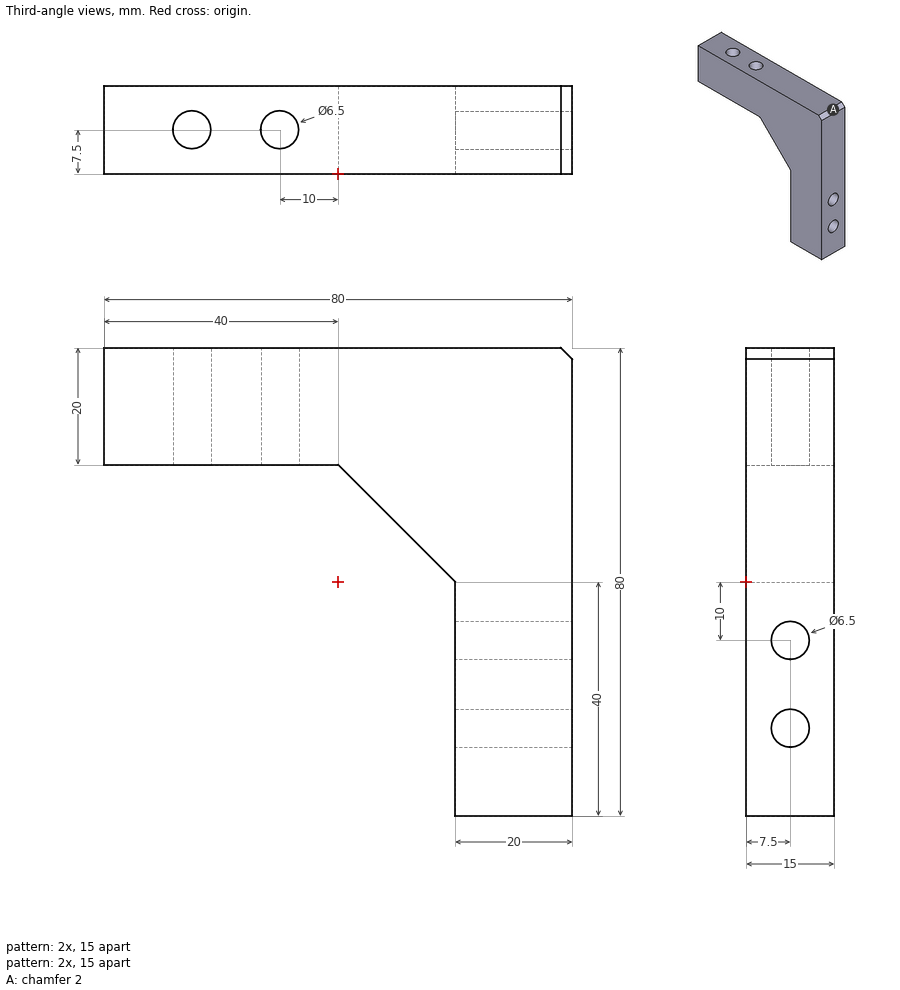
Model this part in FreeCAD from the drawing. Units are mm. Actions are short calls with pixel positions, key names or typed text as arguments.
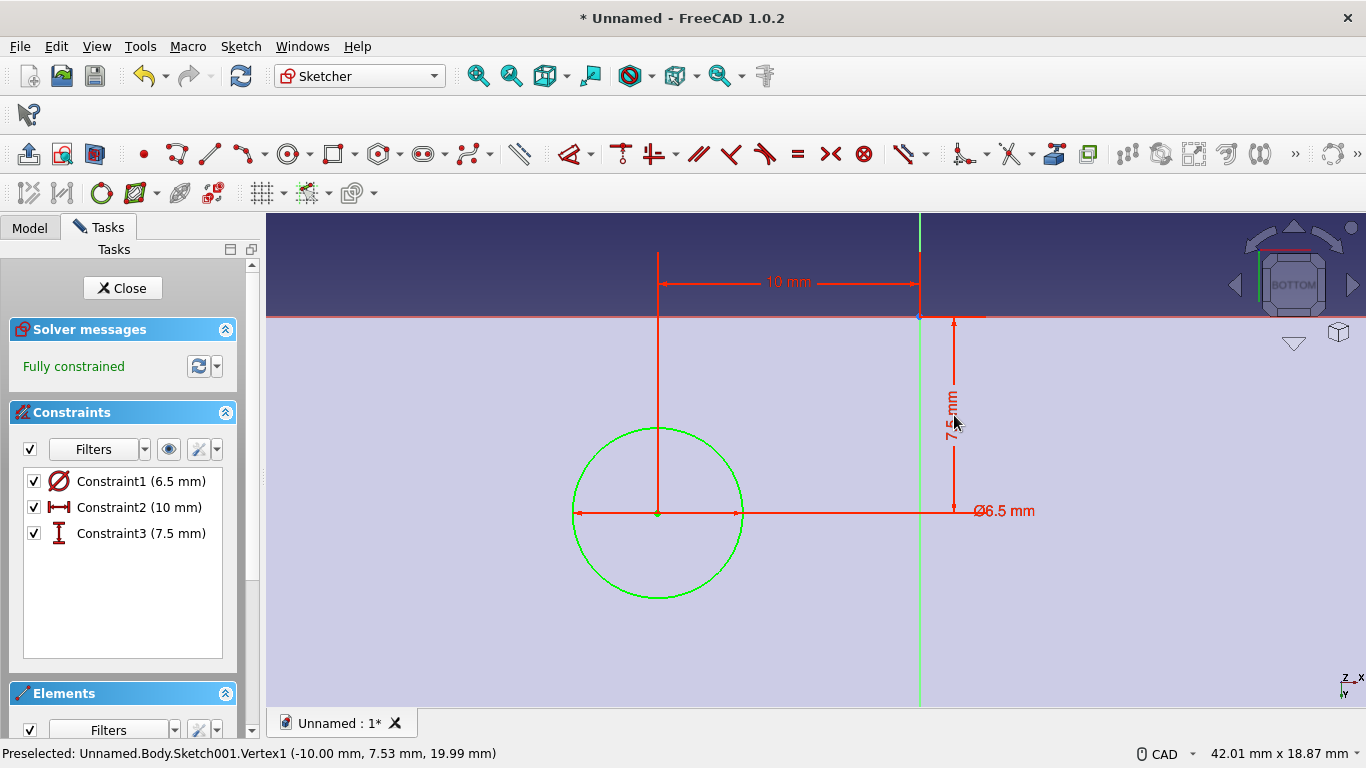
click(123, 288)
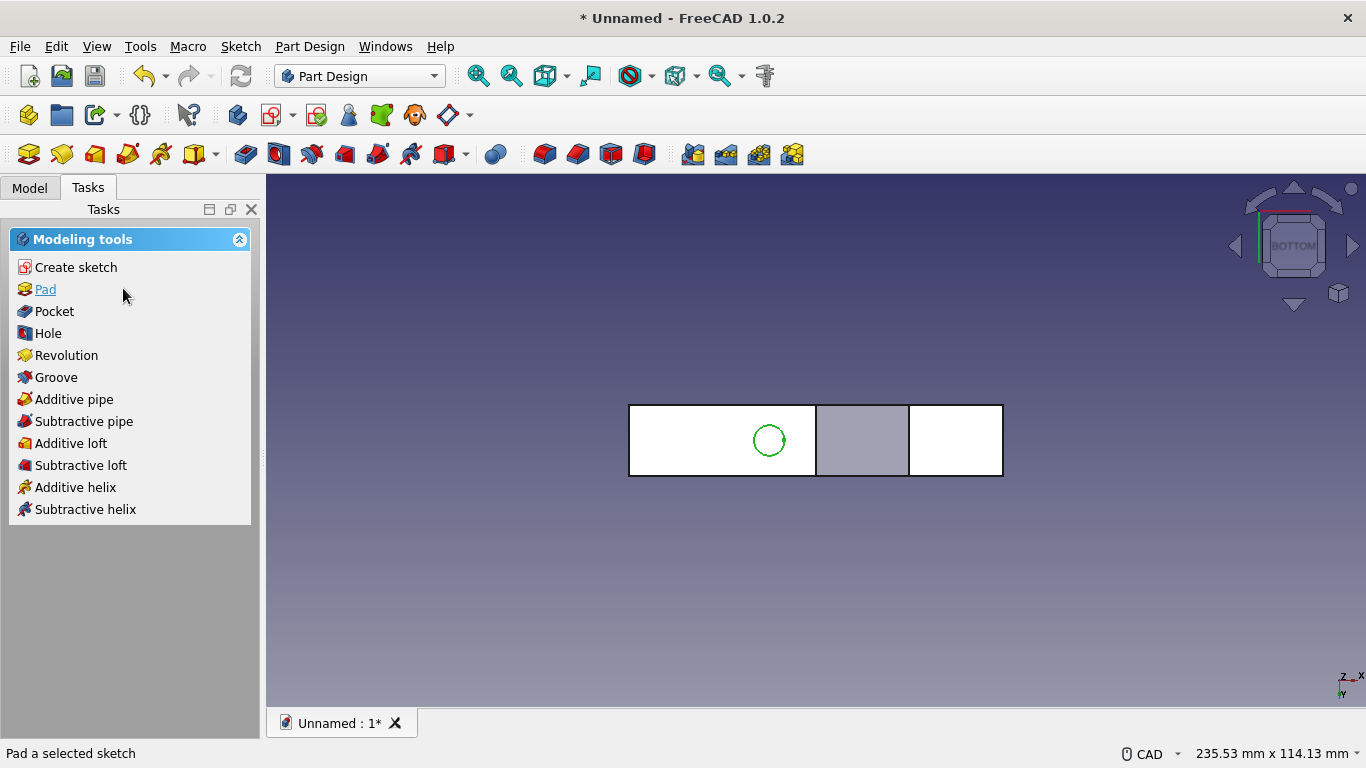
click(246, 154)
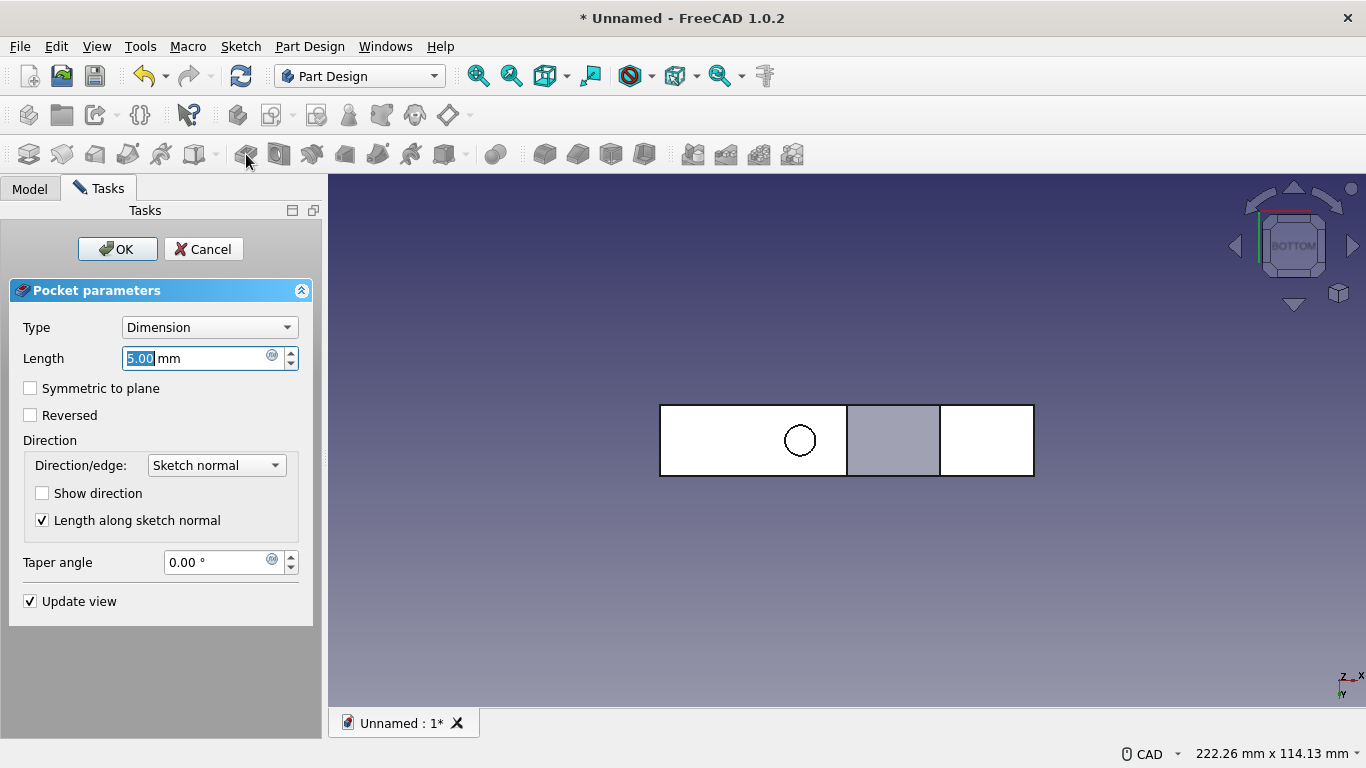
click(210, 328)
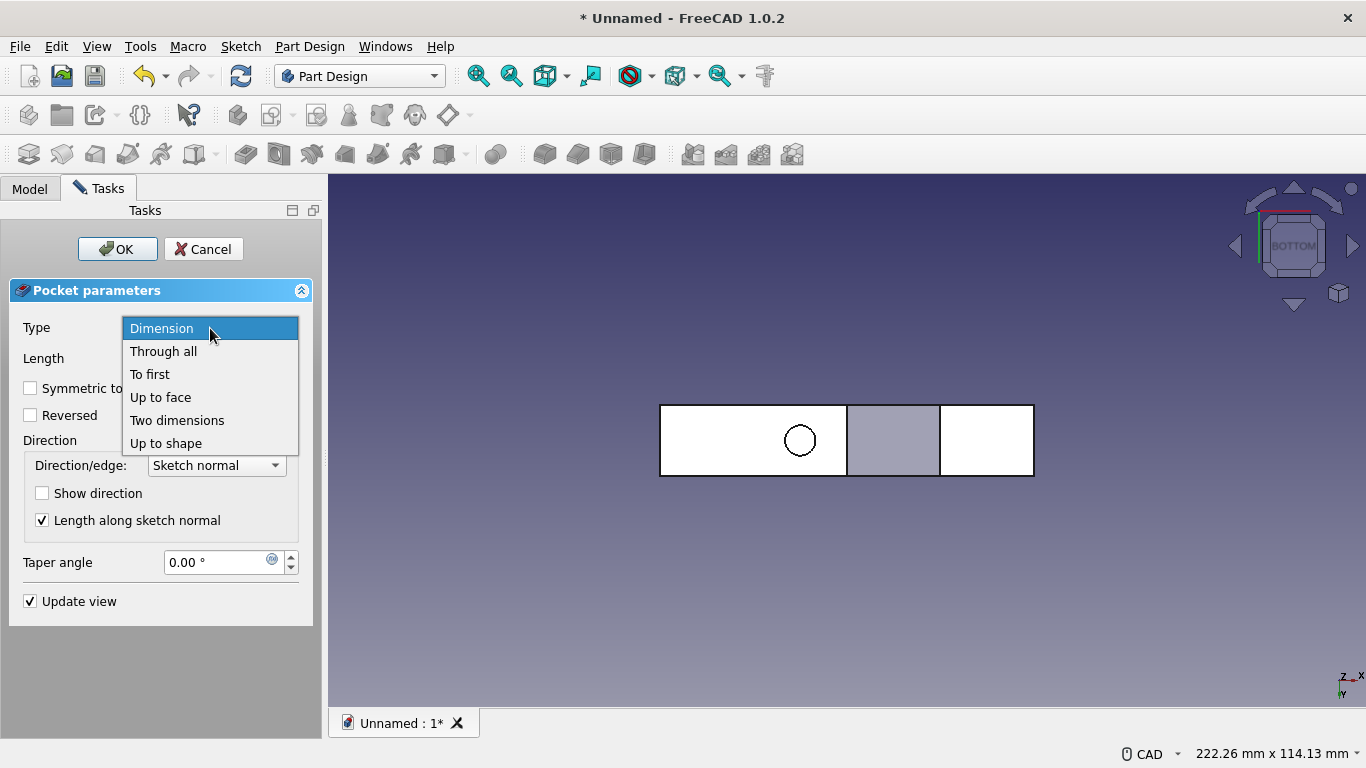
click(208, 352)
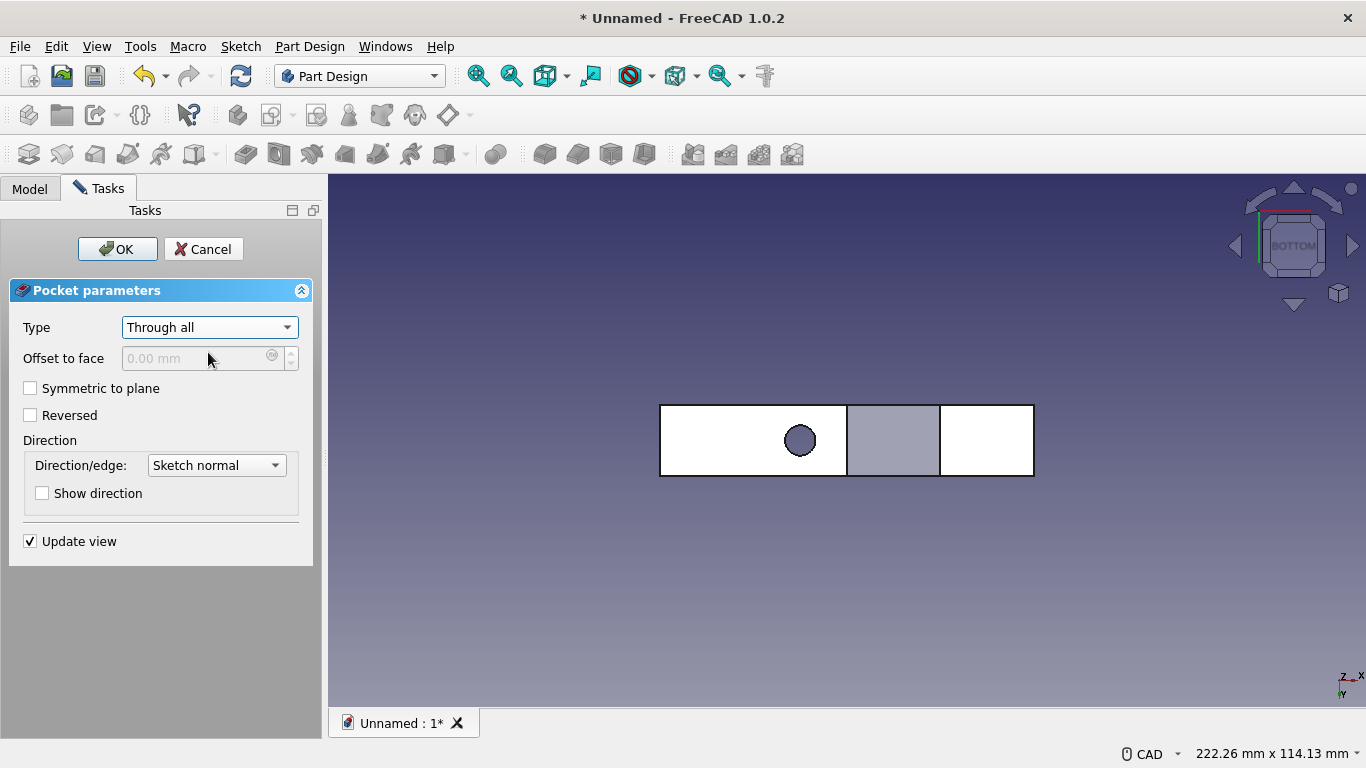
click(118, 249)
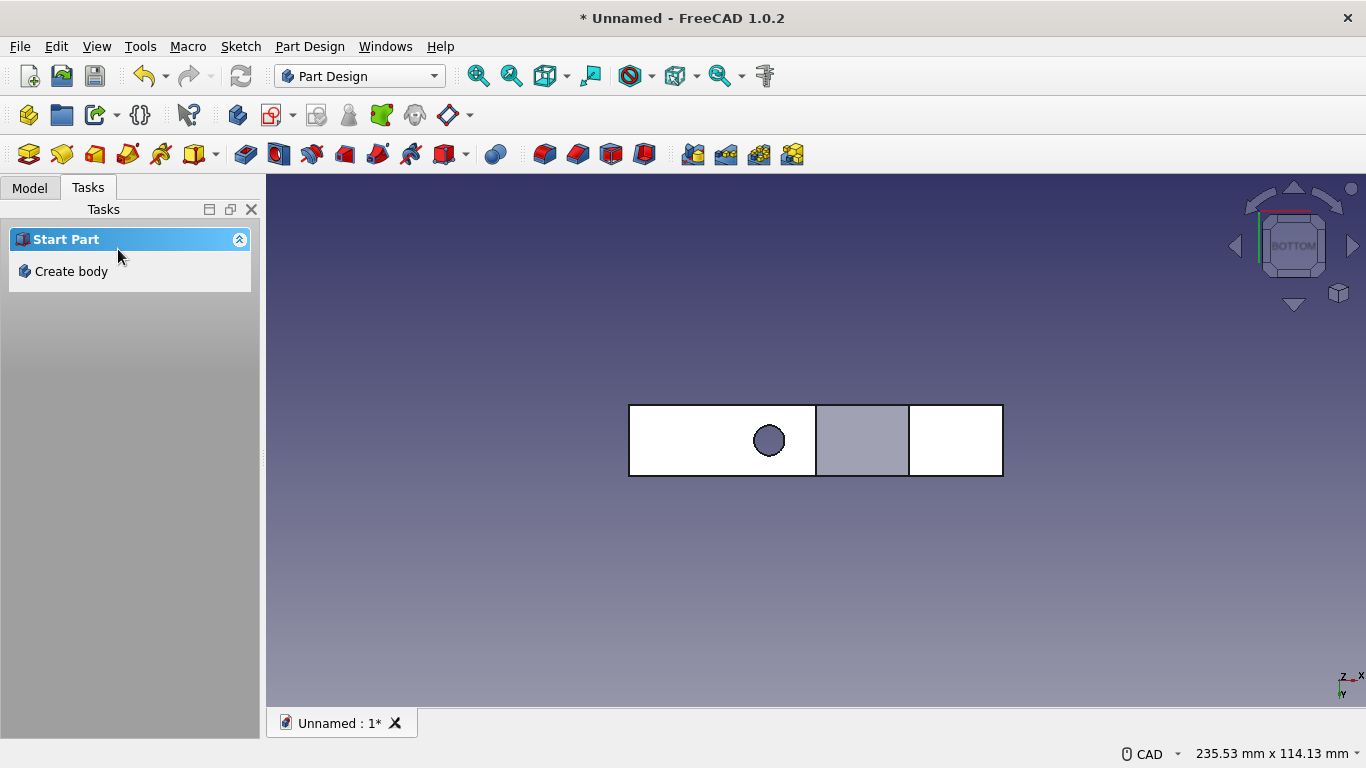
click(479, 76)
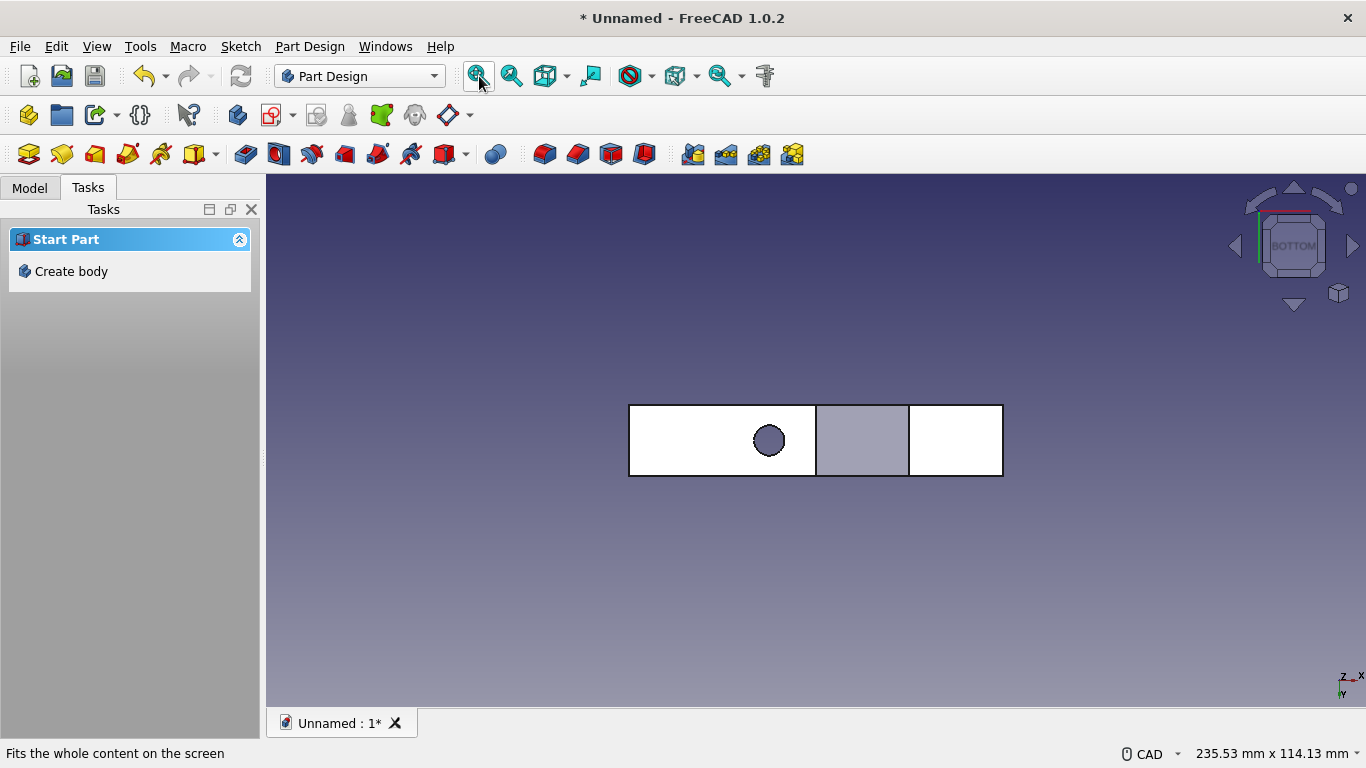
click(30, 188)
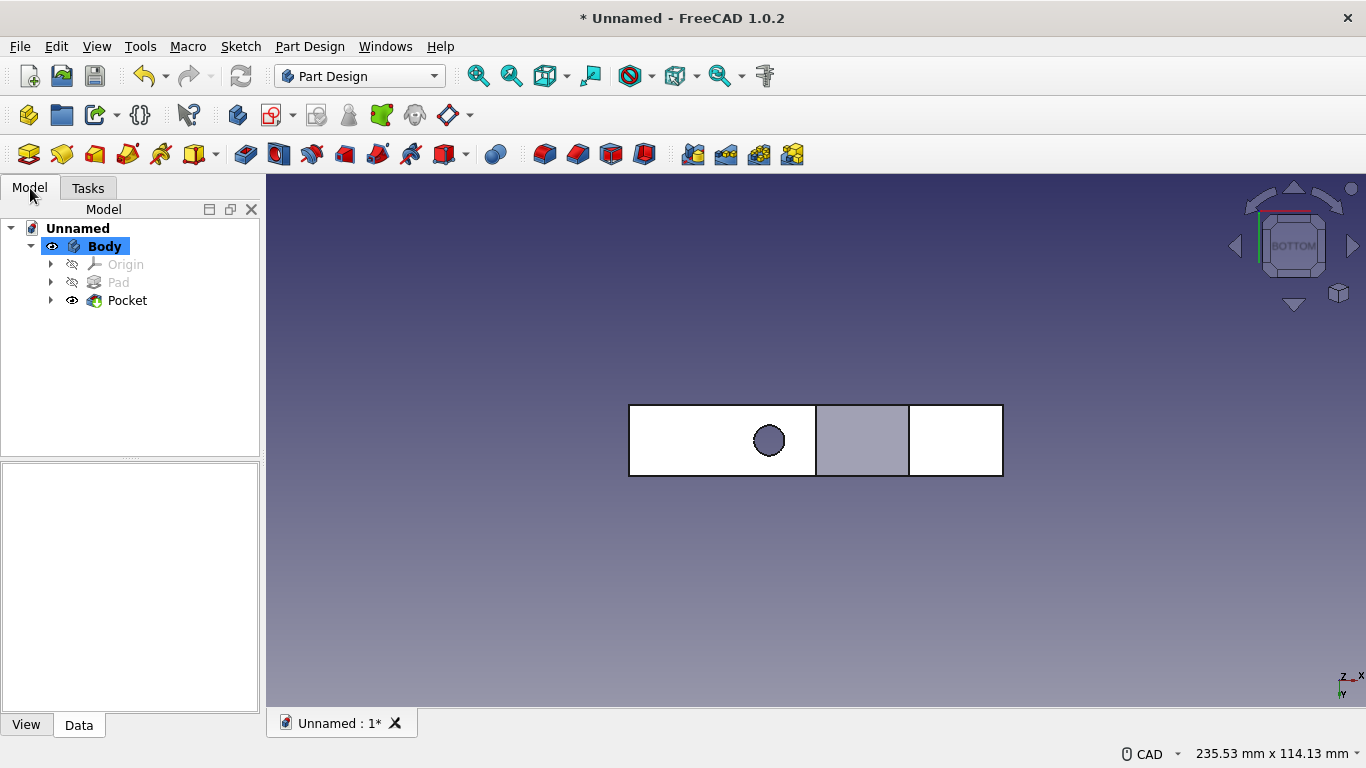
click(117, 300)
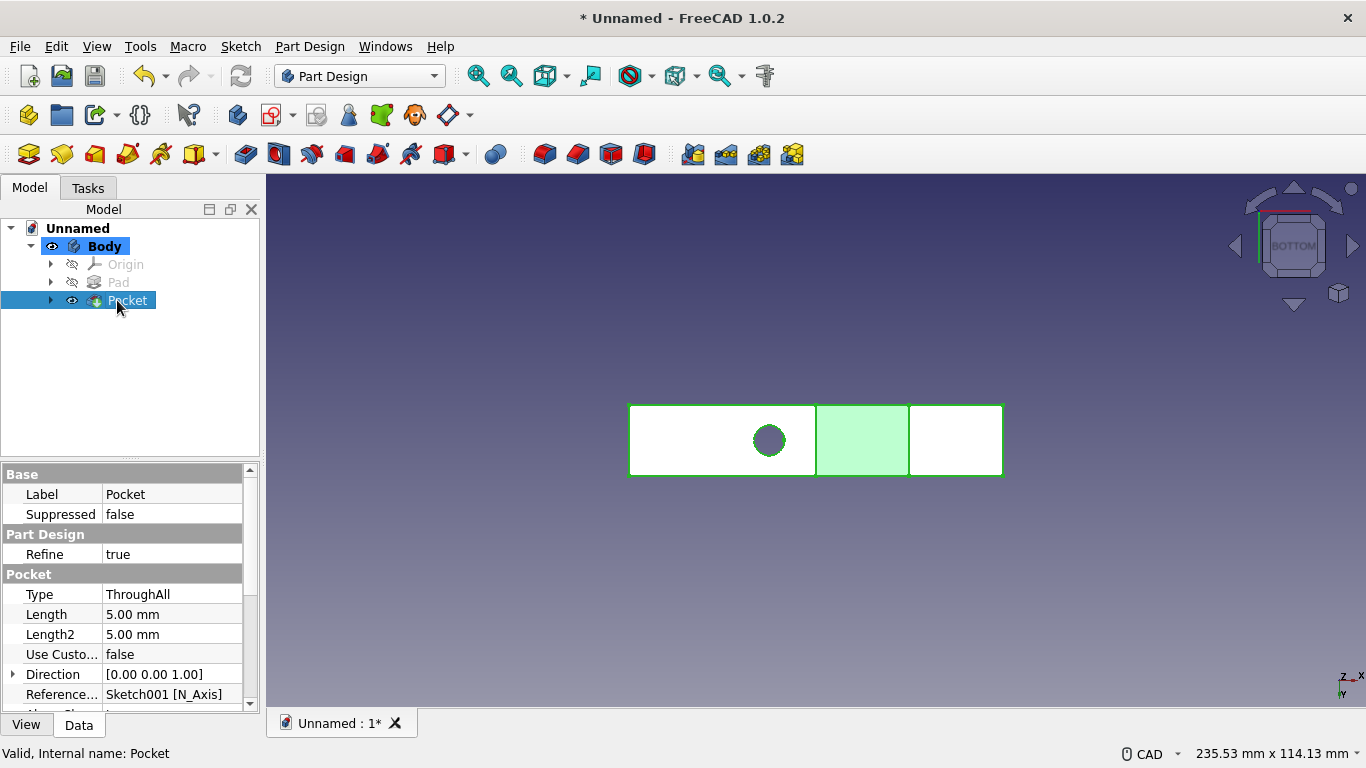
click(726, 154)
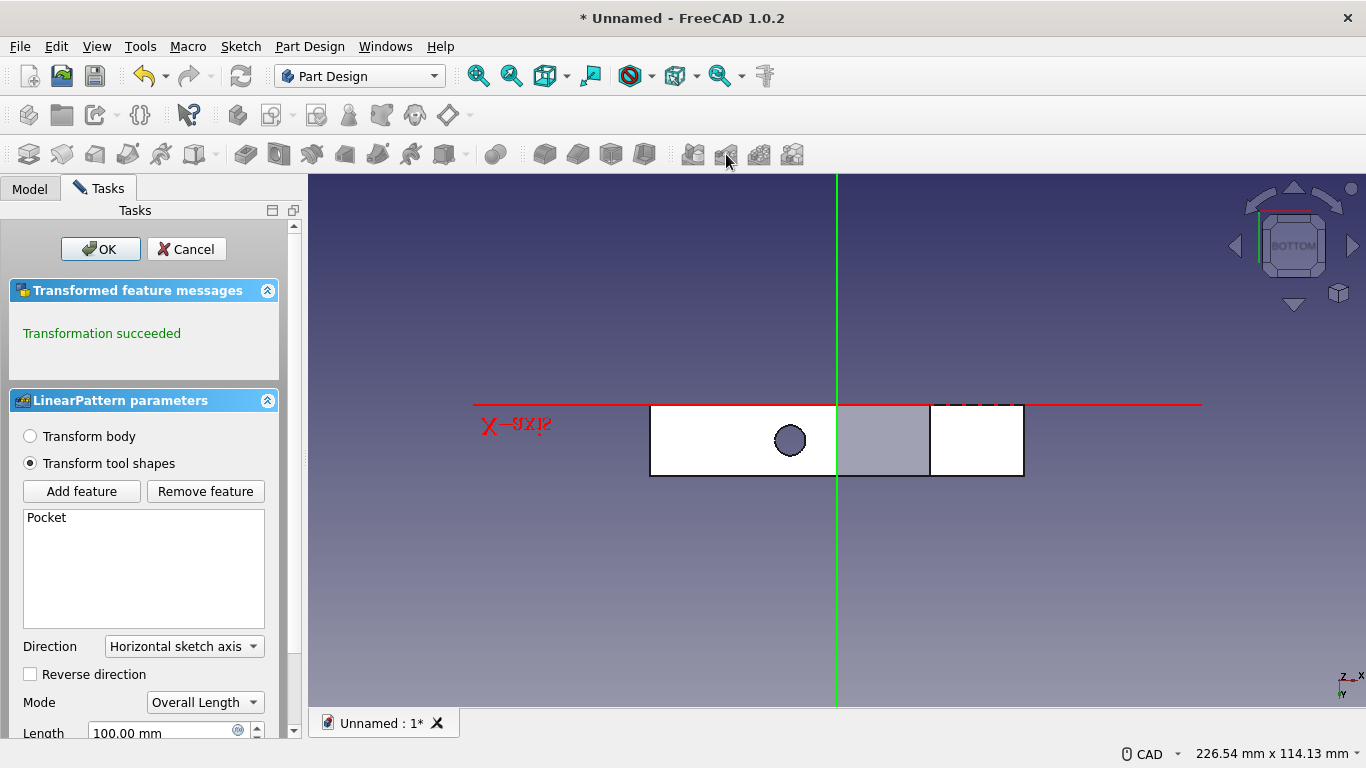
click(185, 646)